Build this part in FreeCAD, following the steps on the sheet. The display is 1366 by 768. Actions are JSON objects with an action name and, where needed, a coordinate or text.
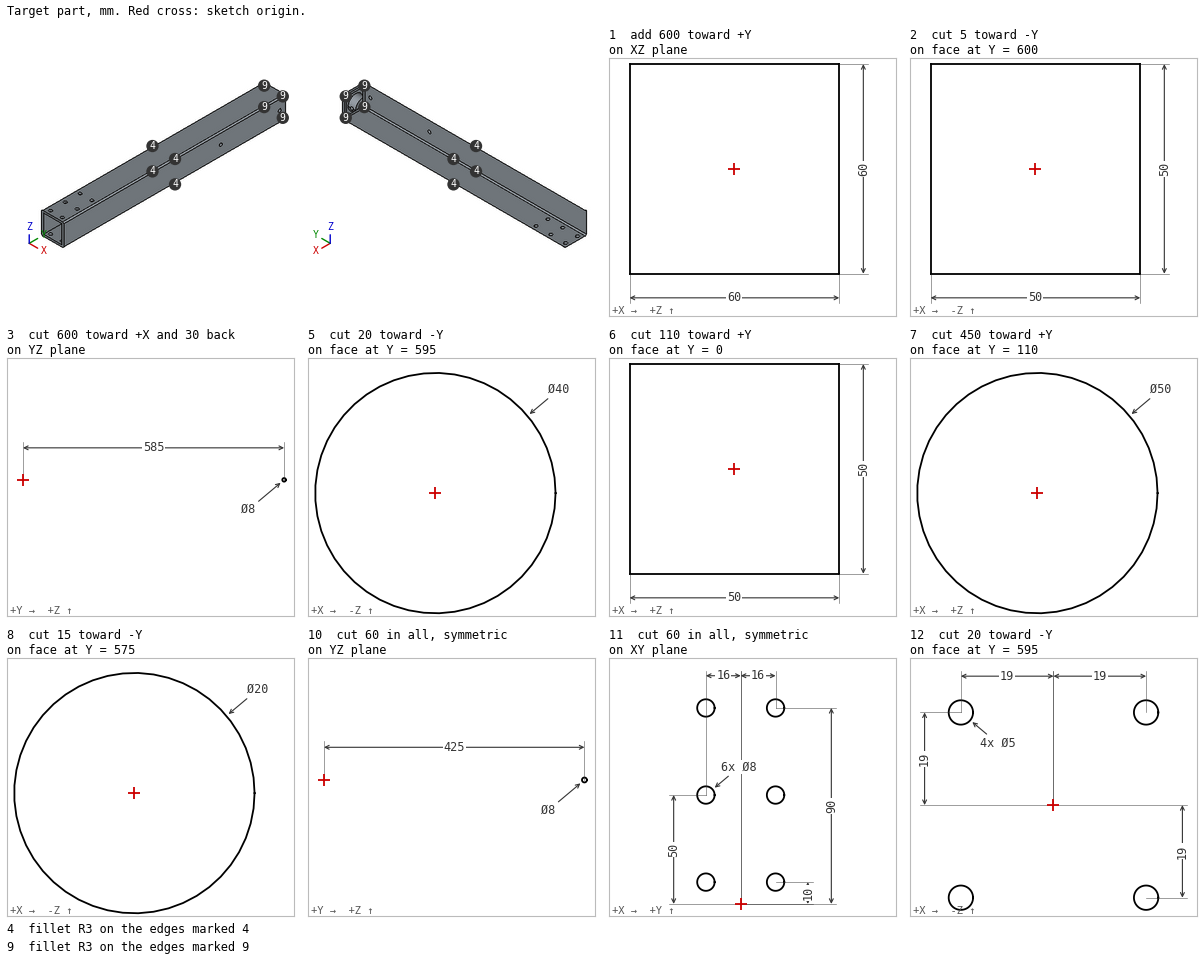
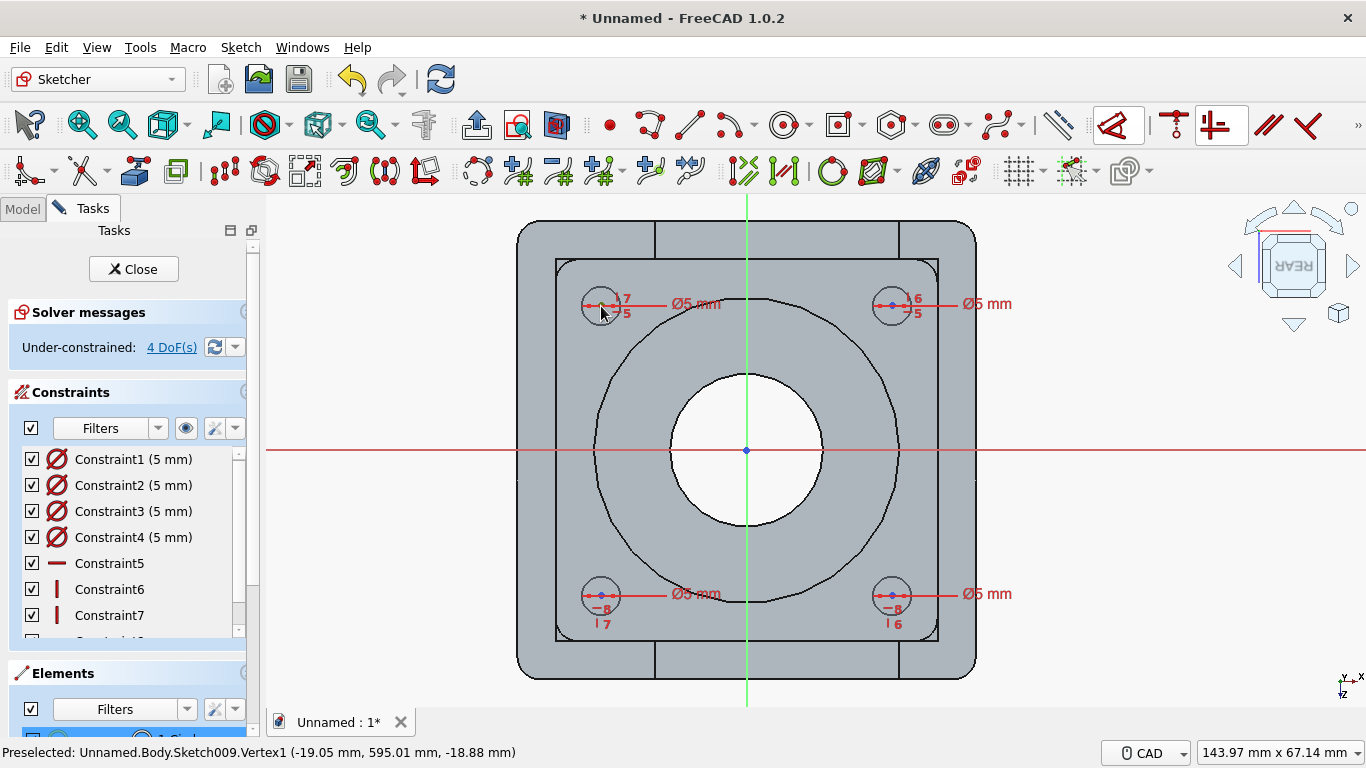
{"action": "left_click", "coordinate": [1138, 126]}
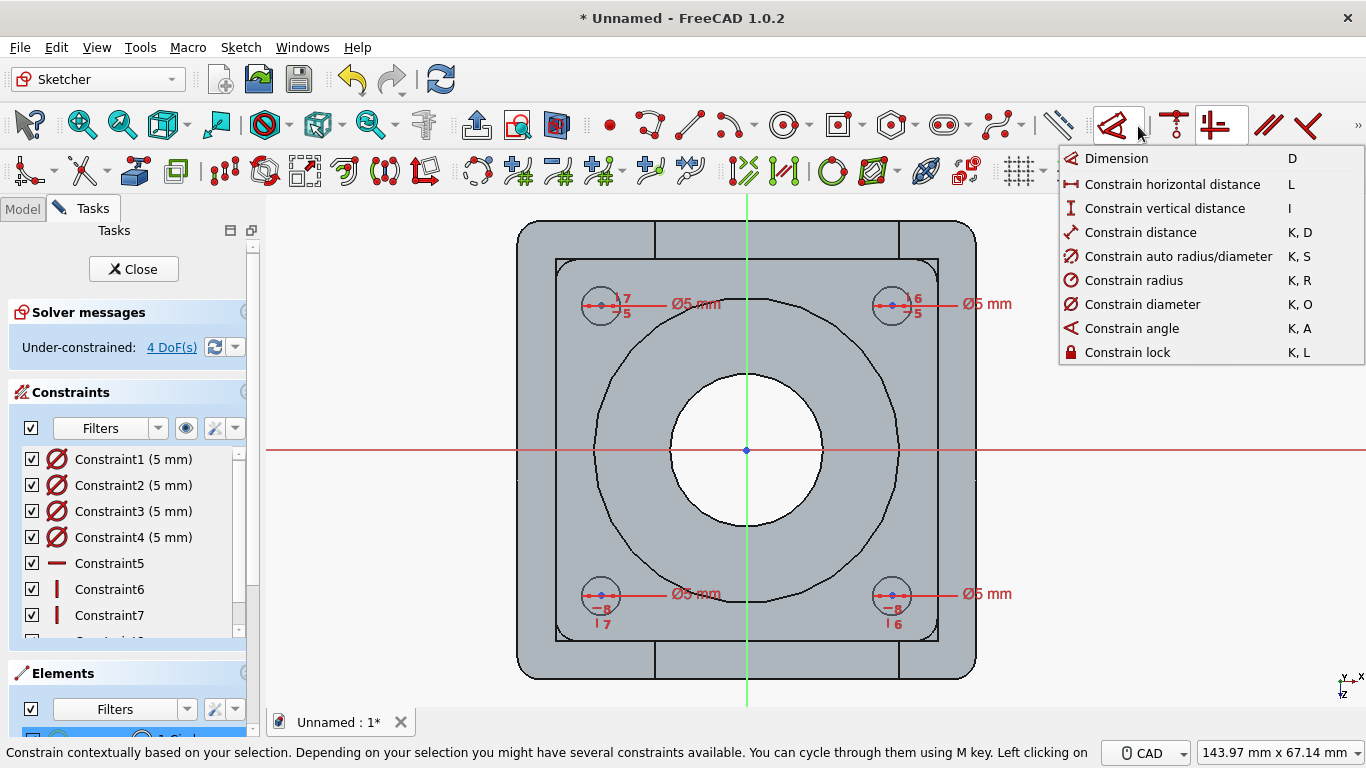
{"action": "left_click", "coordinate": [1212, 184]}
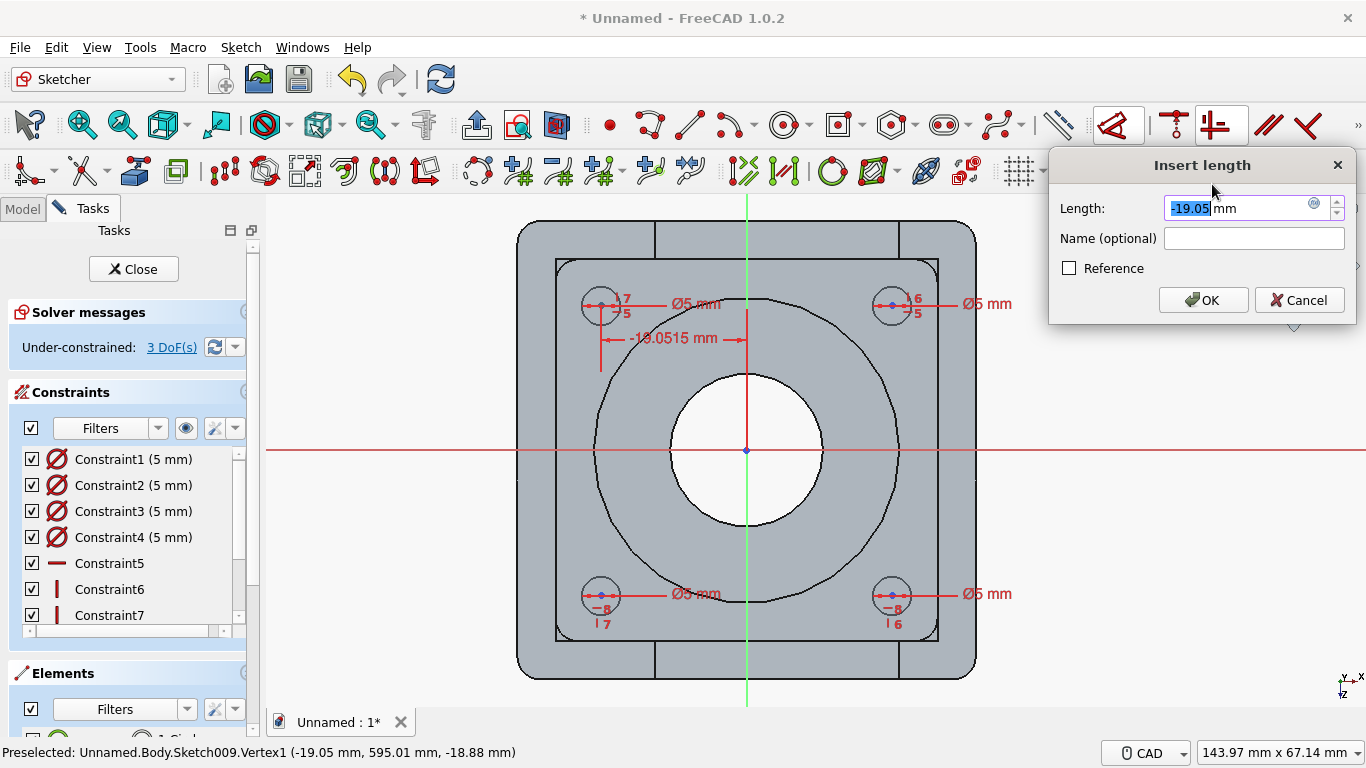
{"action": "type", "text": "-19"}
{"action": "key", "text": "Return"}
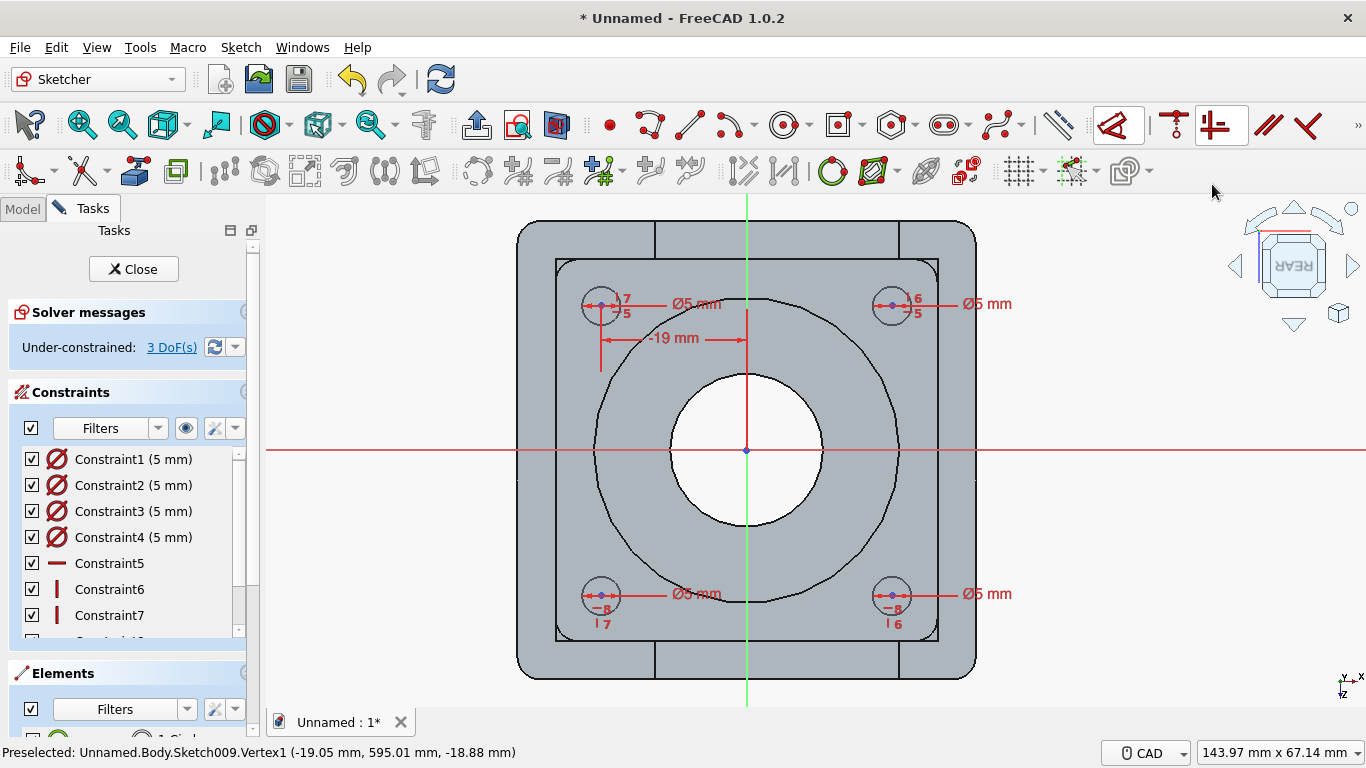
{"action": "left_click", "coordinate": [601, 306]}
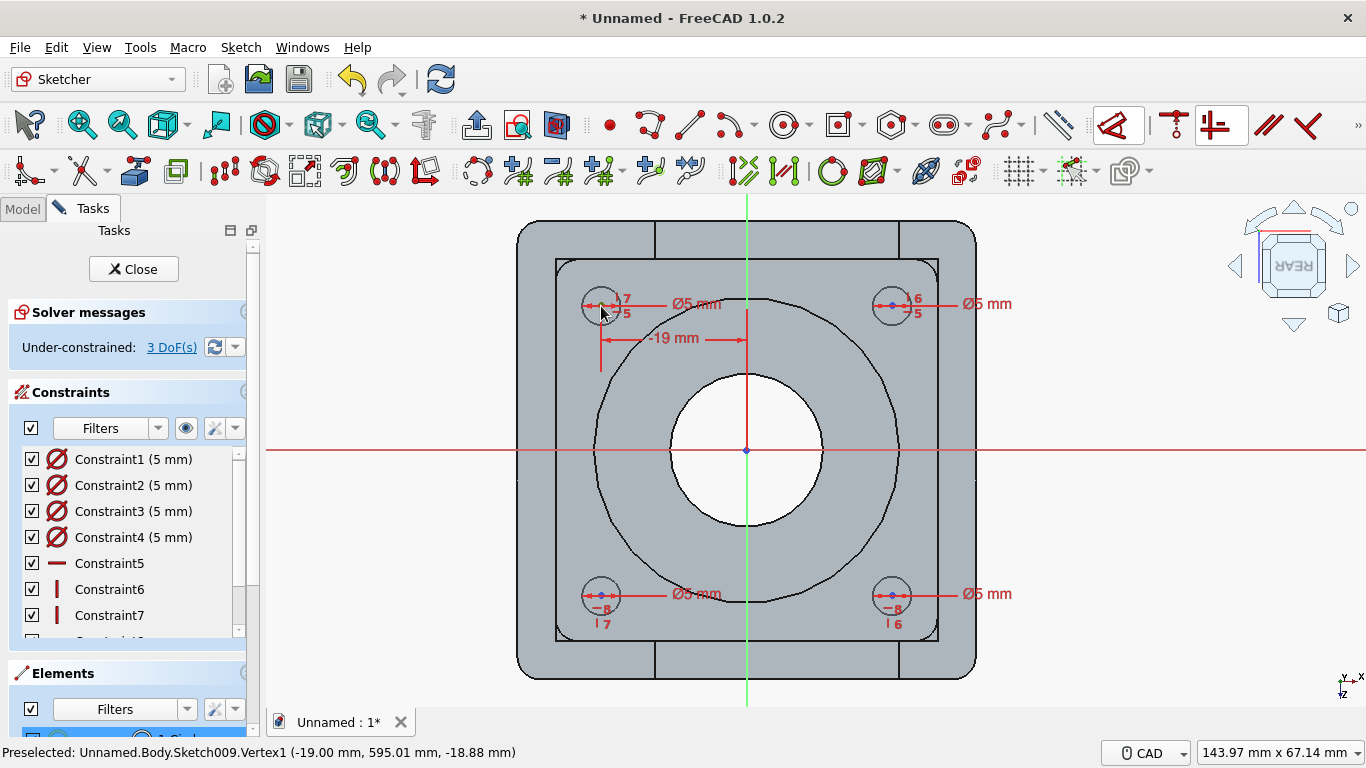
{"action": "key", "text": "i"}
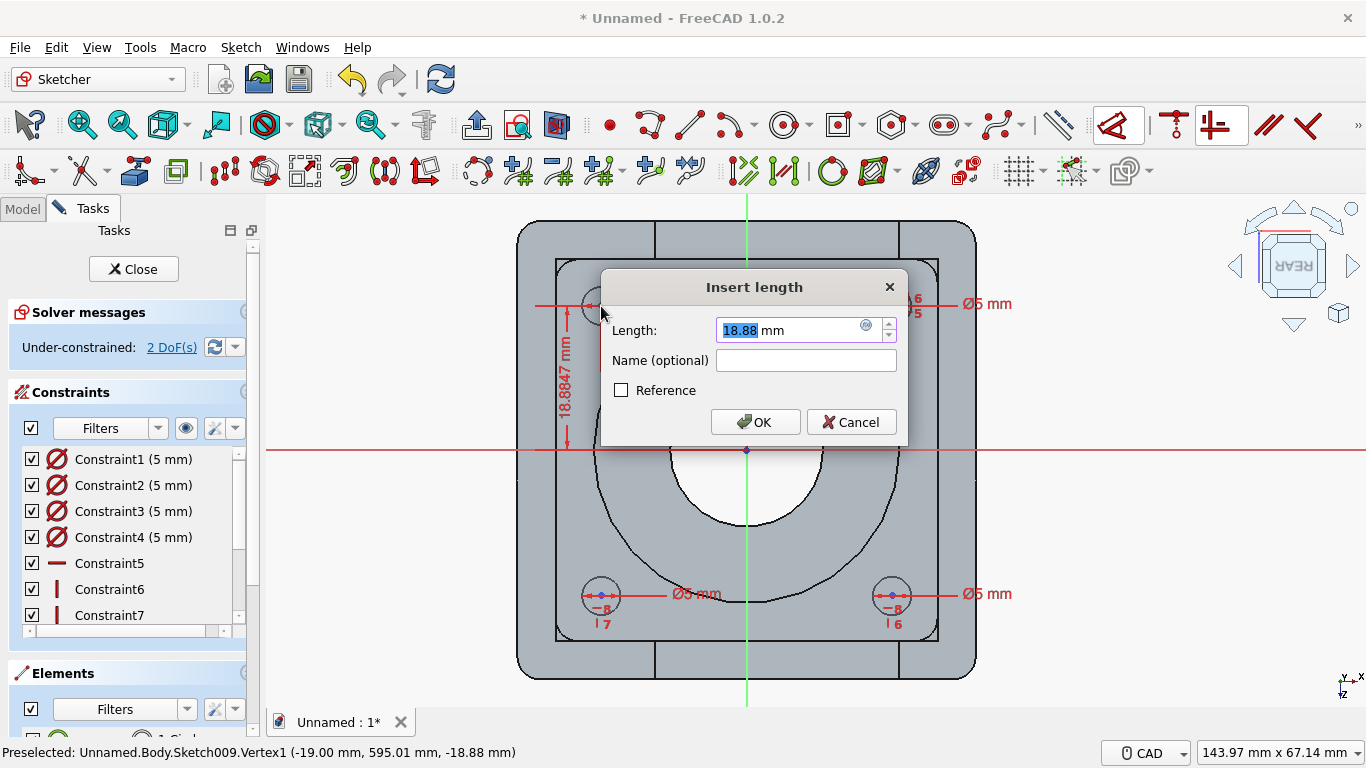
{"action": "type", "text": "19"}
{"action": "key", "text": "Return"}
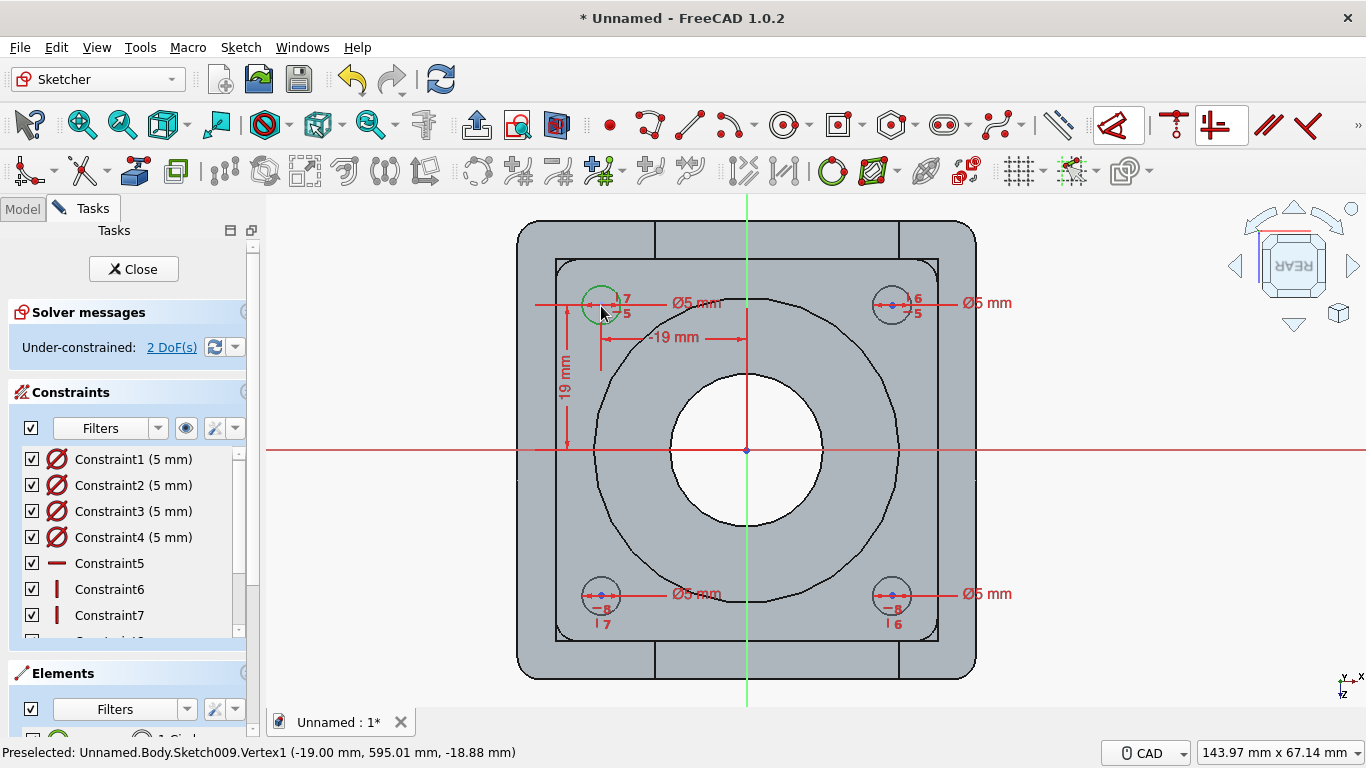
{"action": "left_click", "coordinate": [892, 305]}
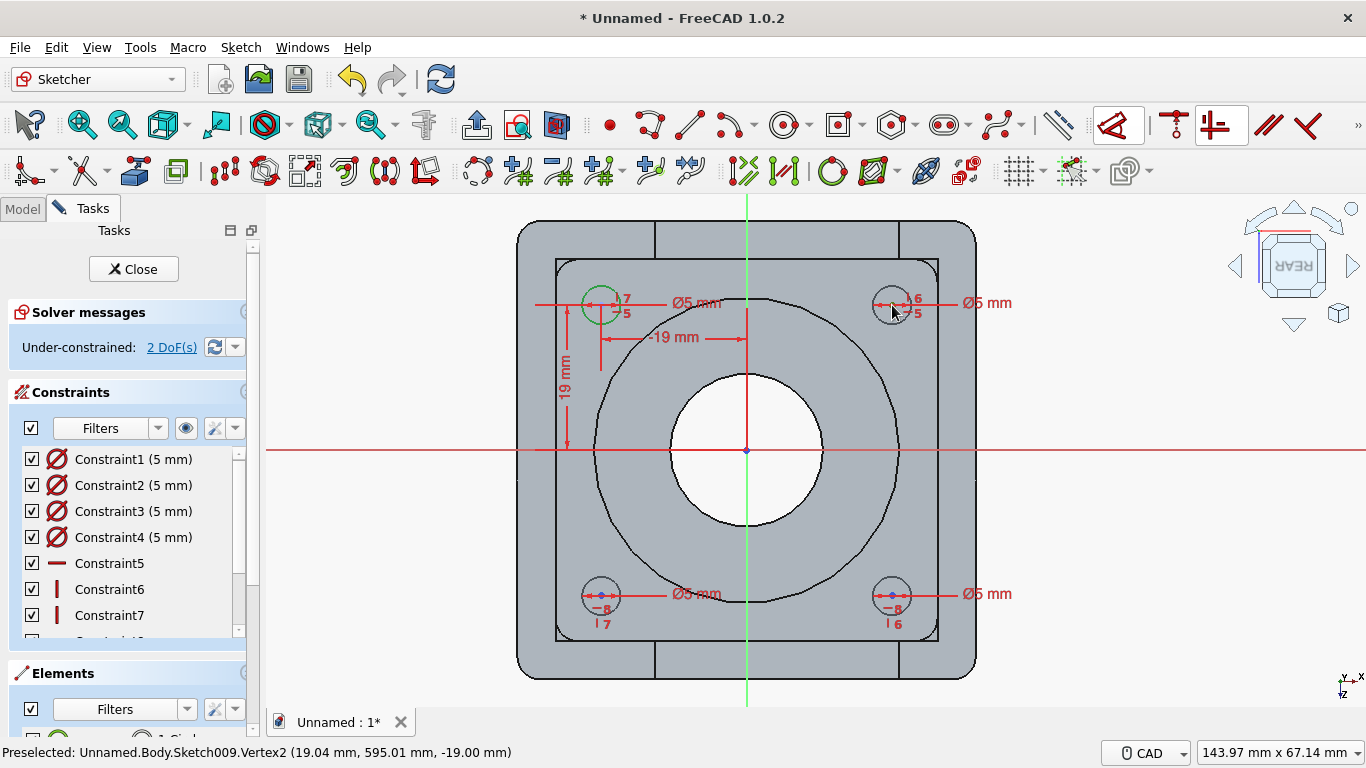
{"action": "key", "text": "l"}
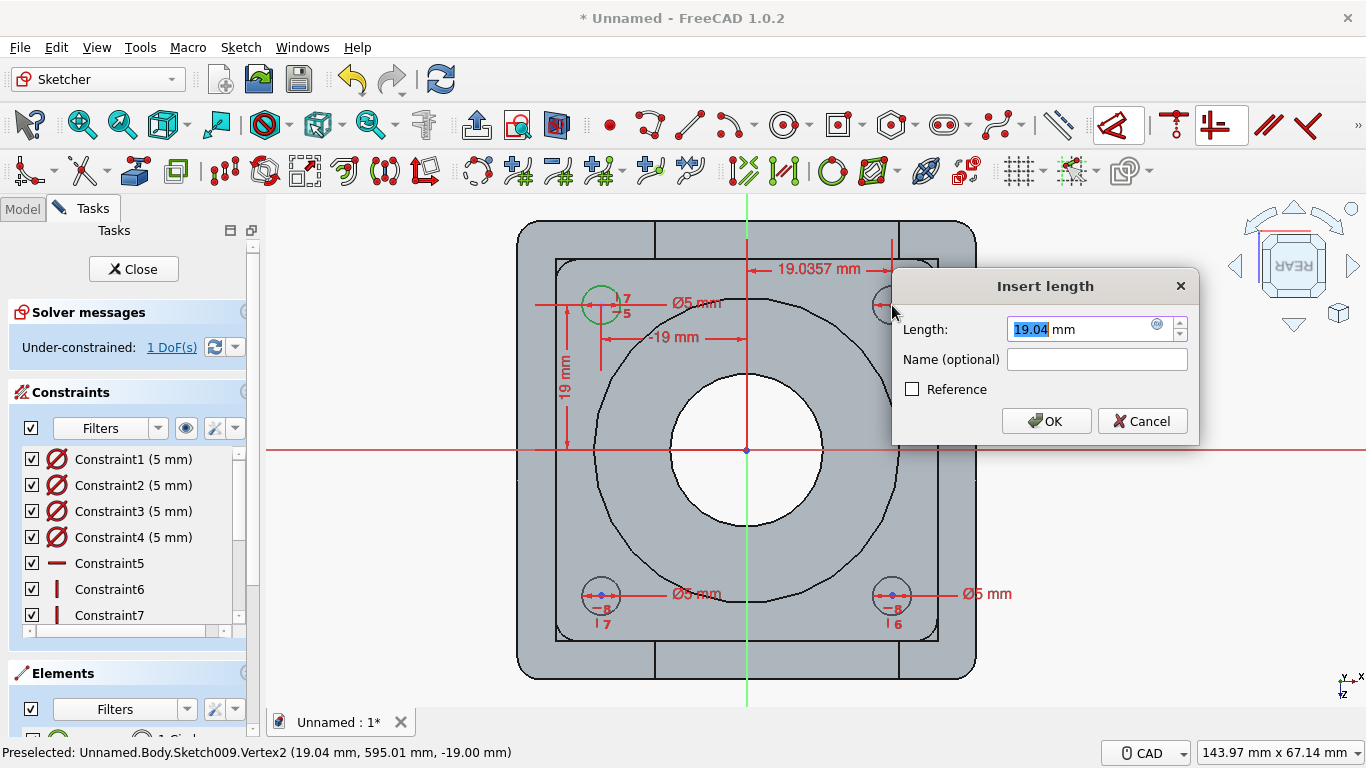
{"action": "type", "text": "19"}
{"action": "key", "text": "Return"}